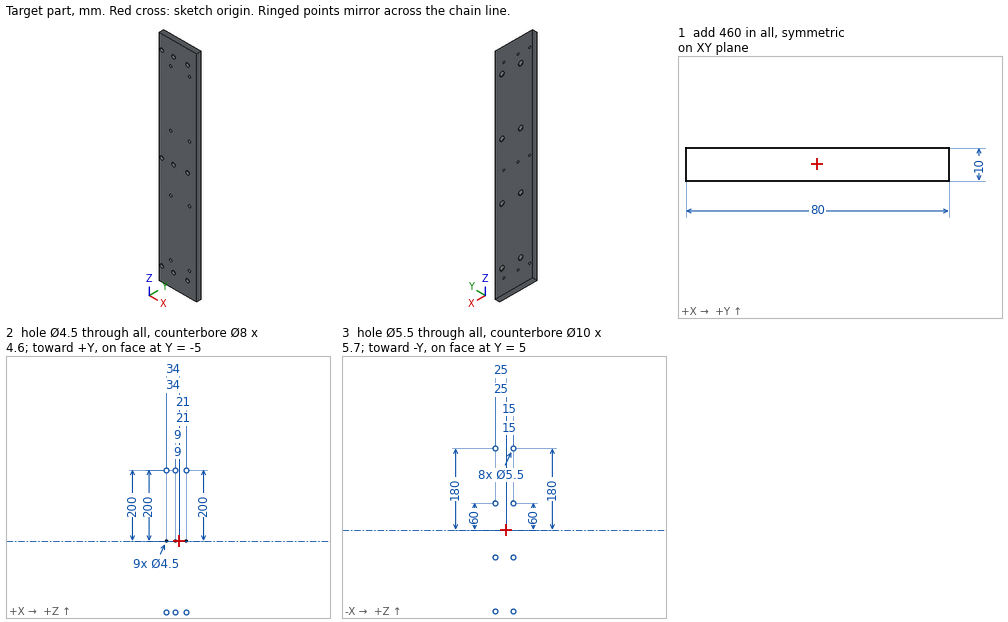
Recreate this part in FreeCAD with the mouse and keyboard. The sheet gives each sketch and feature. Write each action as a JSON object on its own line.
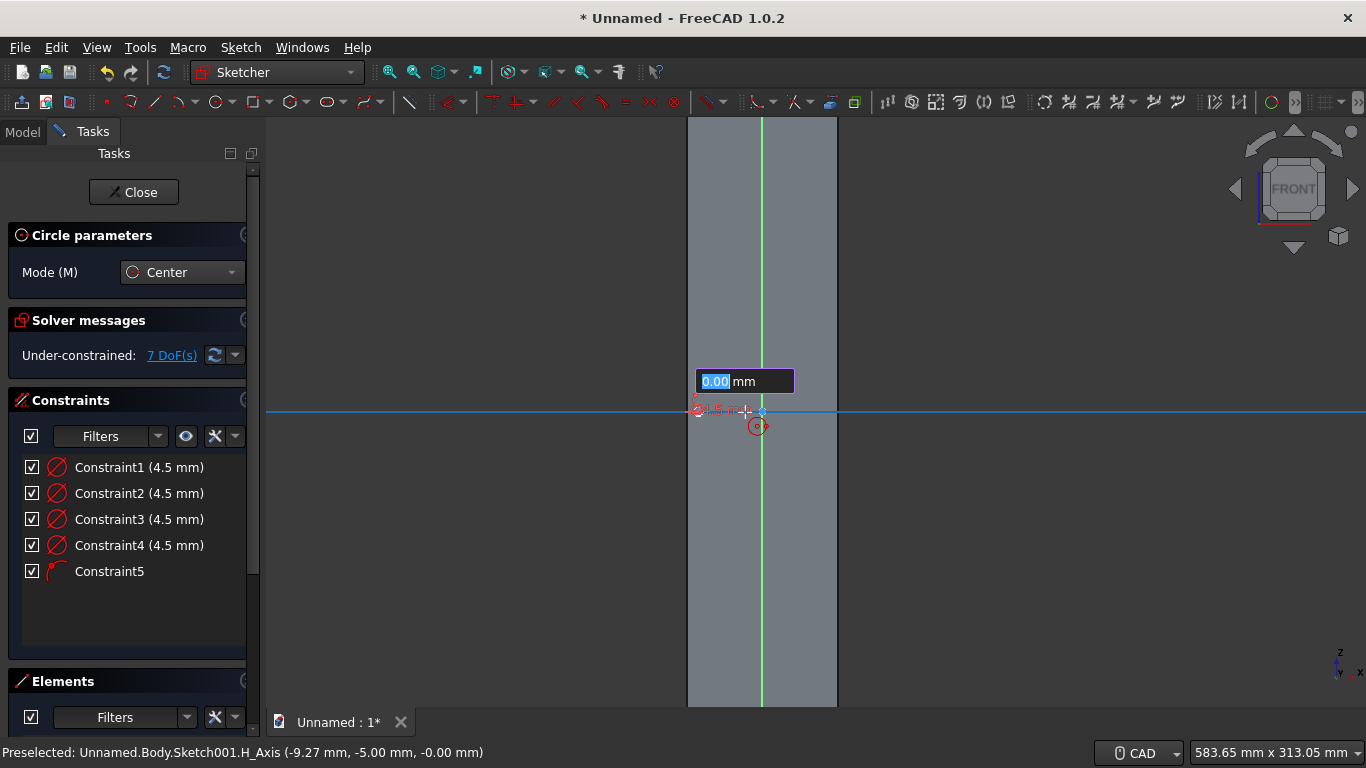
{"action": "scroll", "coordinate": [744, 416], "scroll_direction": "up", "scroll_amount": 7}
{"action": "mouse_move", "coordinate": [743, 414]}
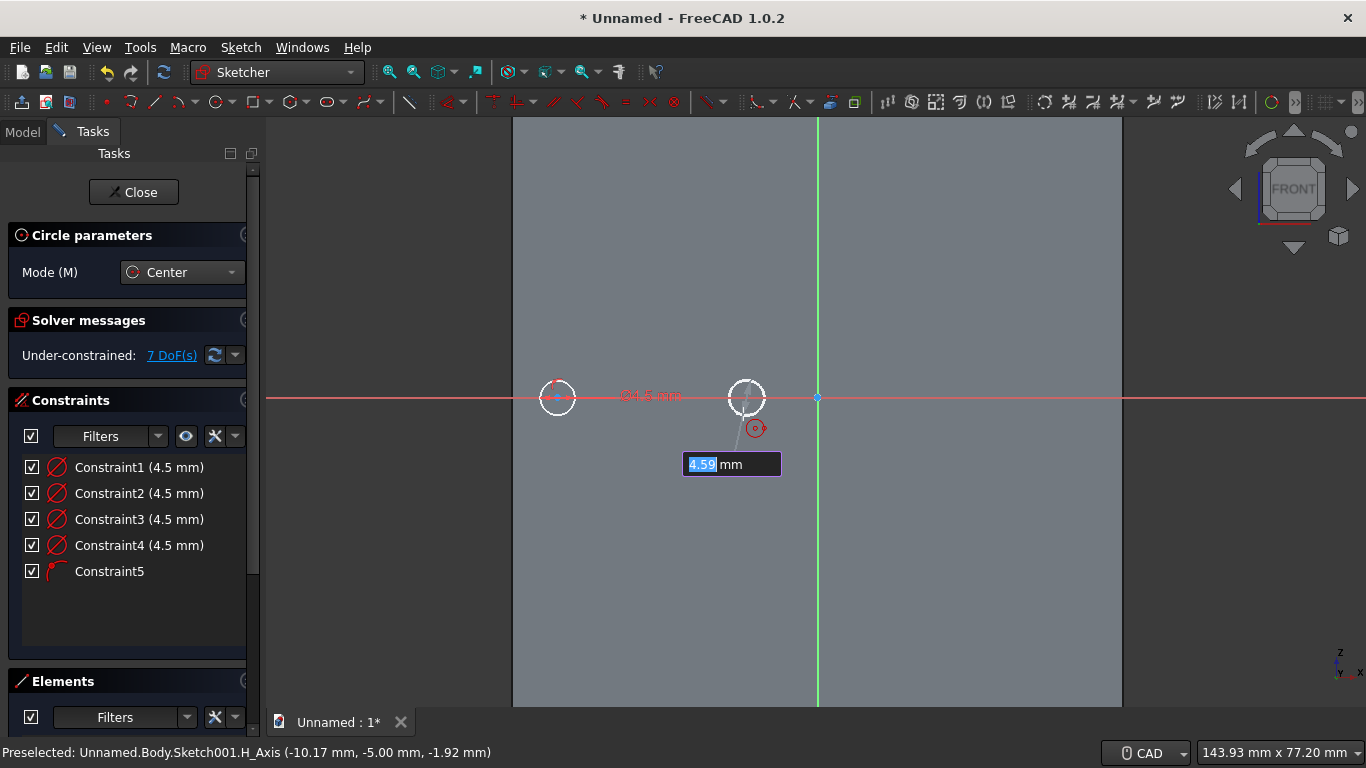
{"action": "type", "text": "4.5"}
{"action": "key", "text": "Return"}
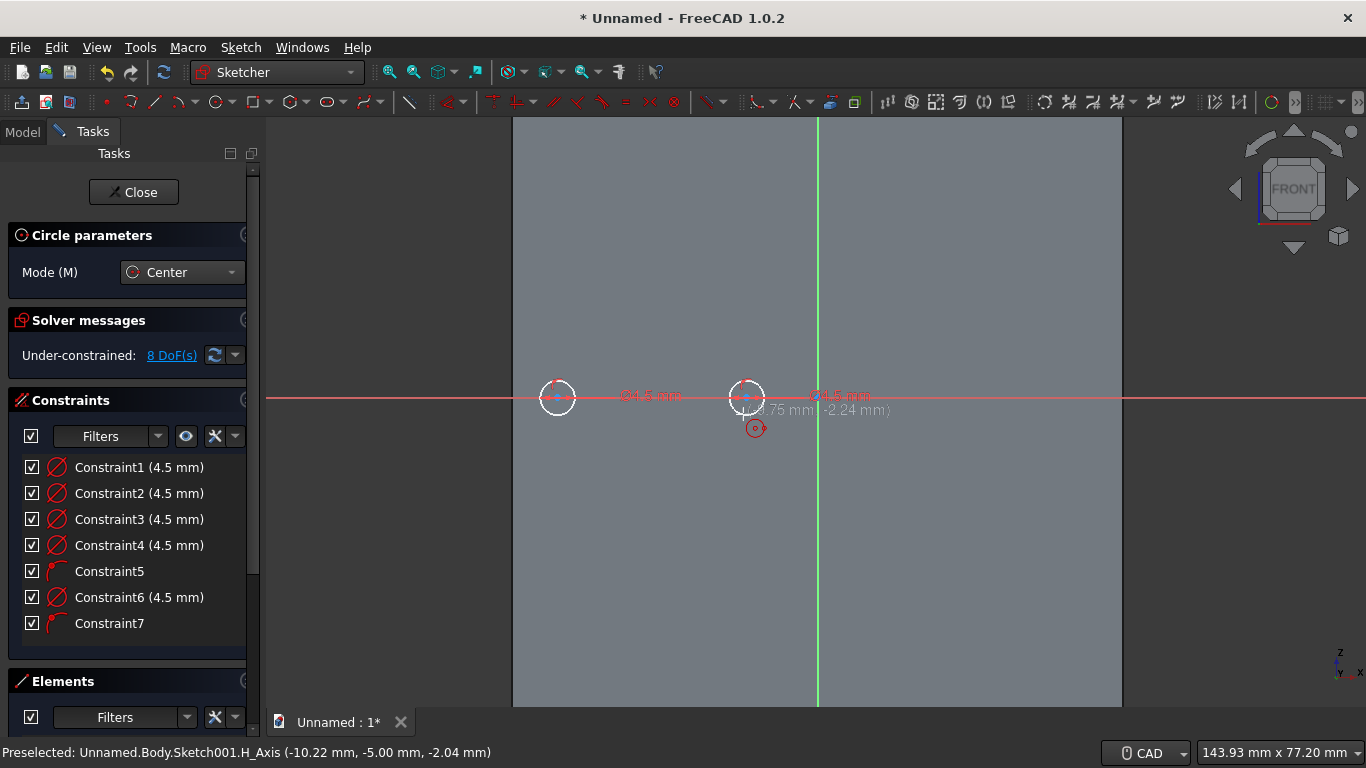
{"action": "scroll", "coordinate": [978, 398], "scroll_direction": "up", "scroll_amount": 2}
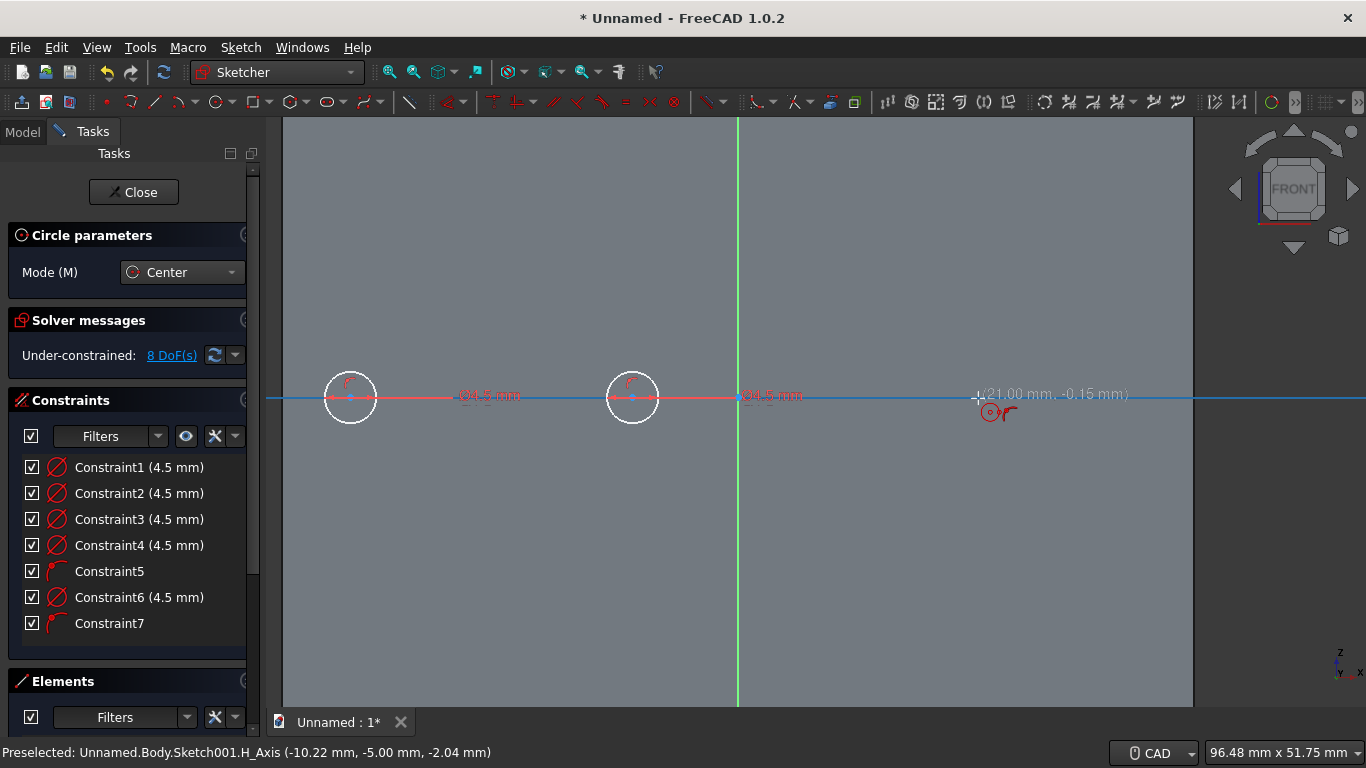
{"action": "scroll", "coordinate": [754, 413], "scroll_direction": "down", "scroll_amount": 13}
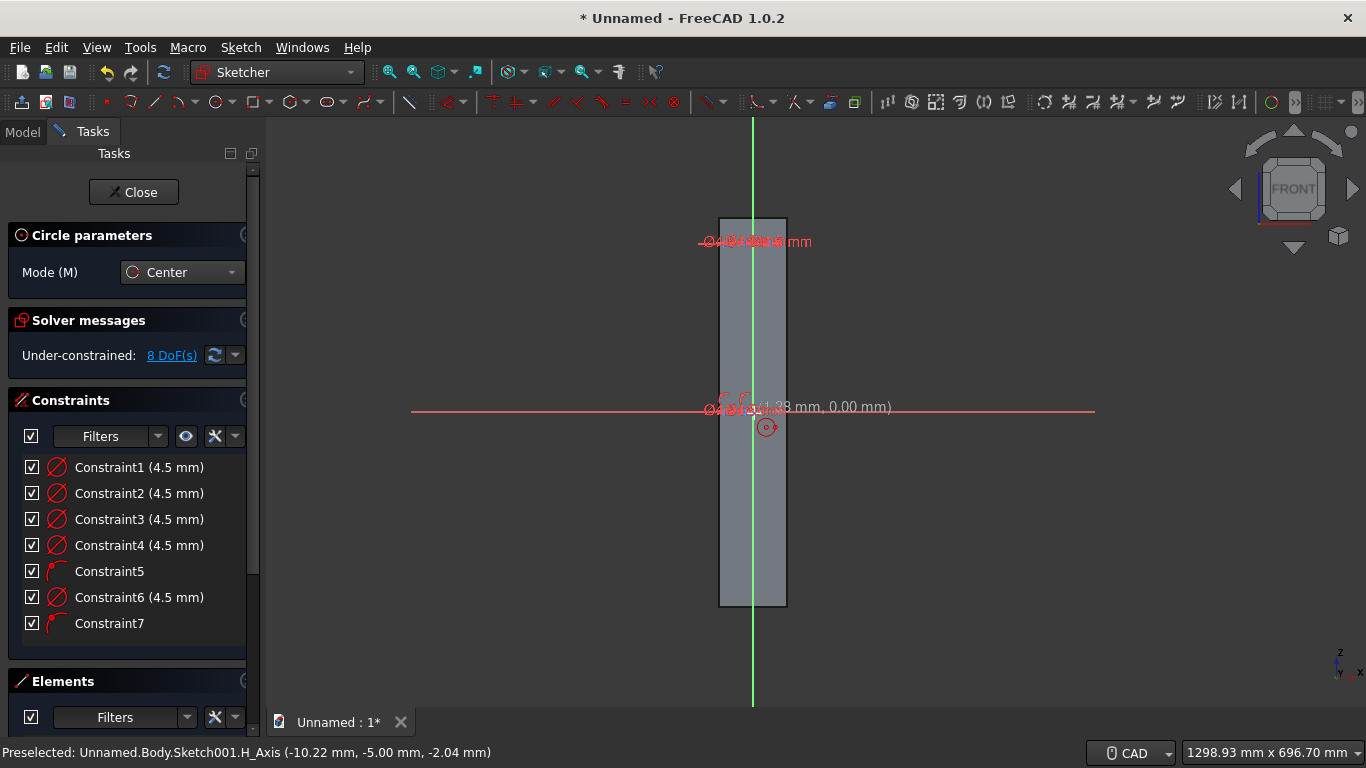
{"action": "left_click", "coordinate": [771, 412]}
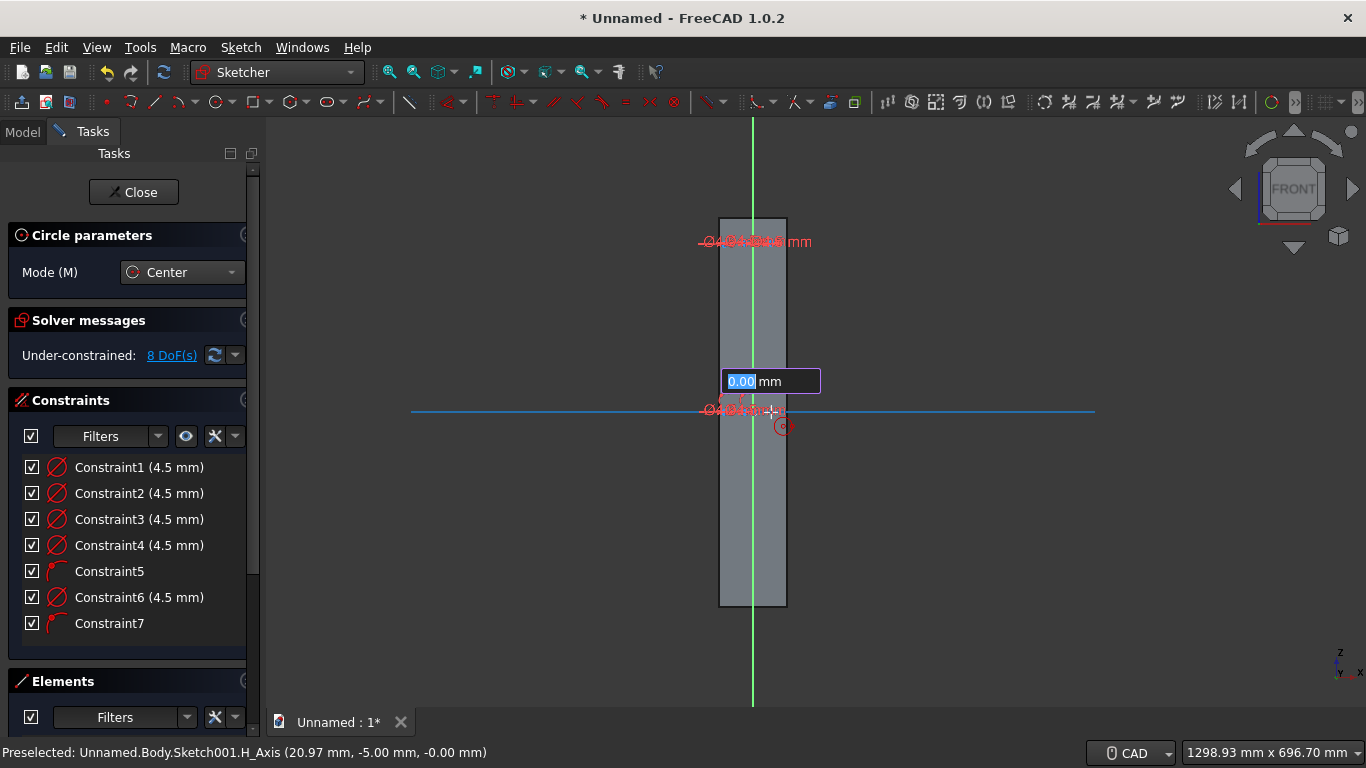
{"action": "scroll", "coordinate": [770, 414], "scroll_direction": "up", "scroll_amount": 11}
{"action": "mouse_move", "coordinate": [770, 411]}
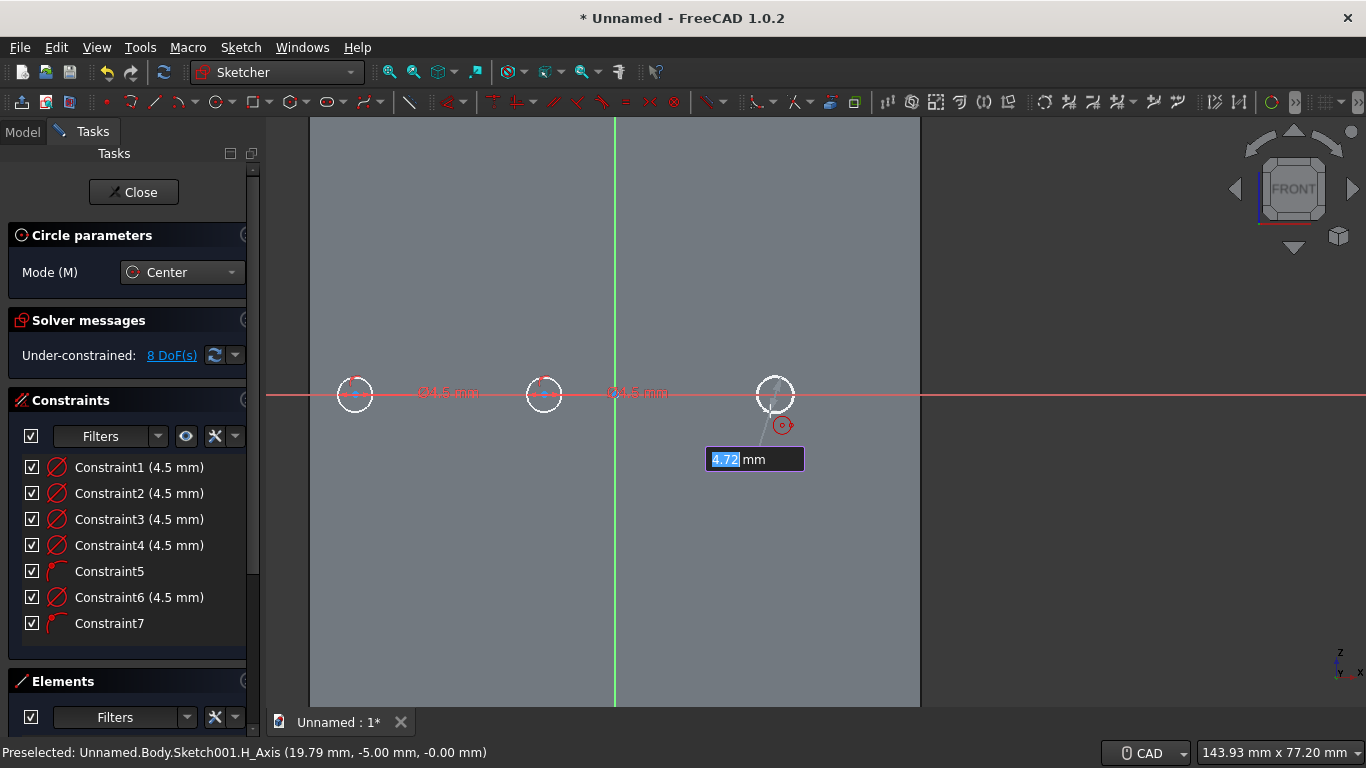
{"action": "type", "text": "4.5"}
{"action": "key", "text": "Return"}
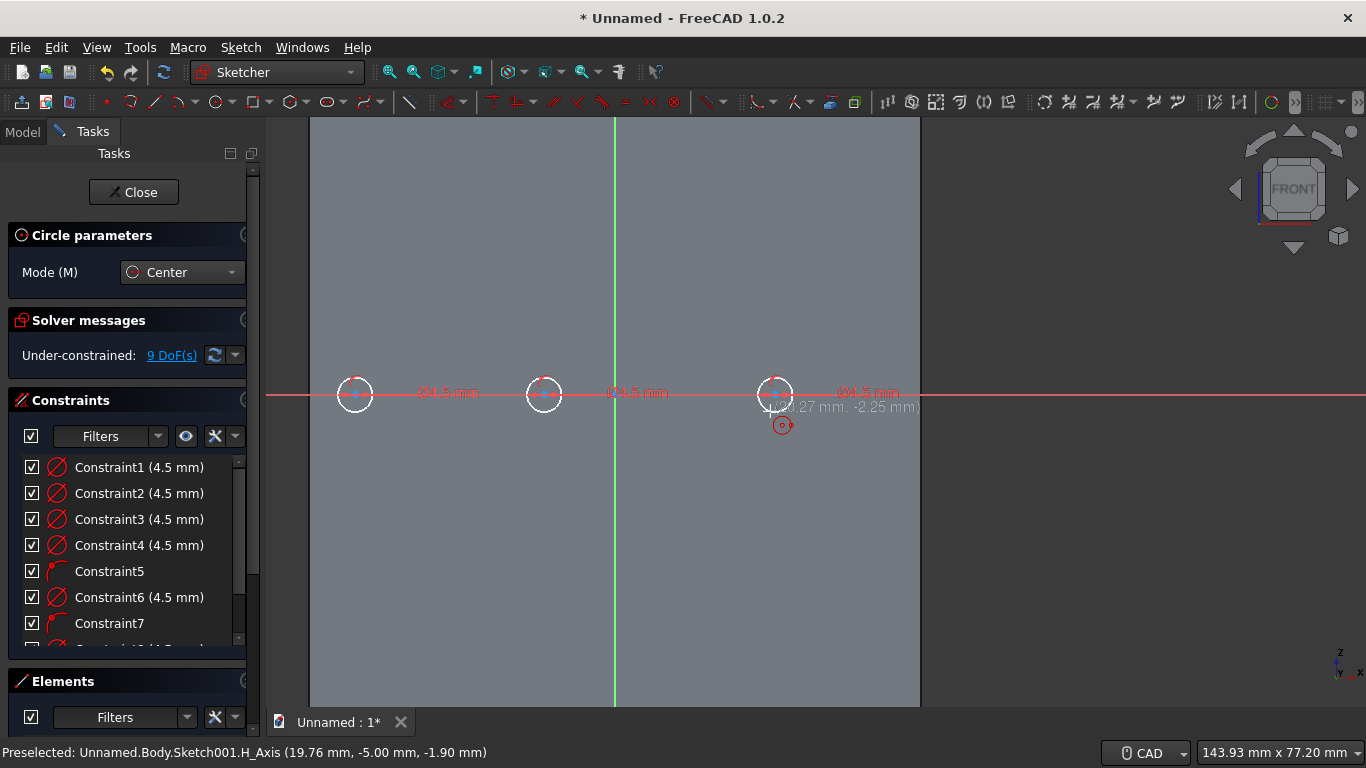
{"action": "scroll", "coordinate": [770, 414], "scroll_direction": "down", "scroll_amount": 11}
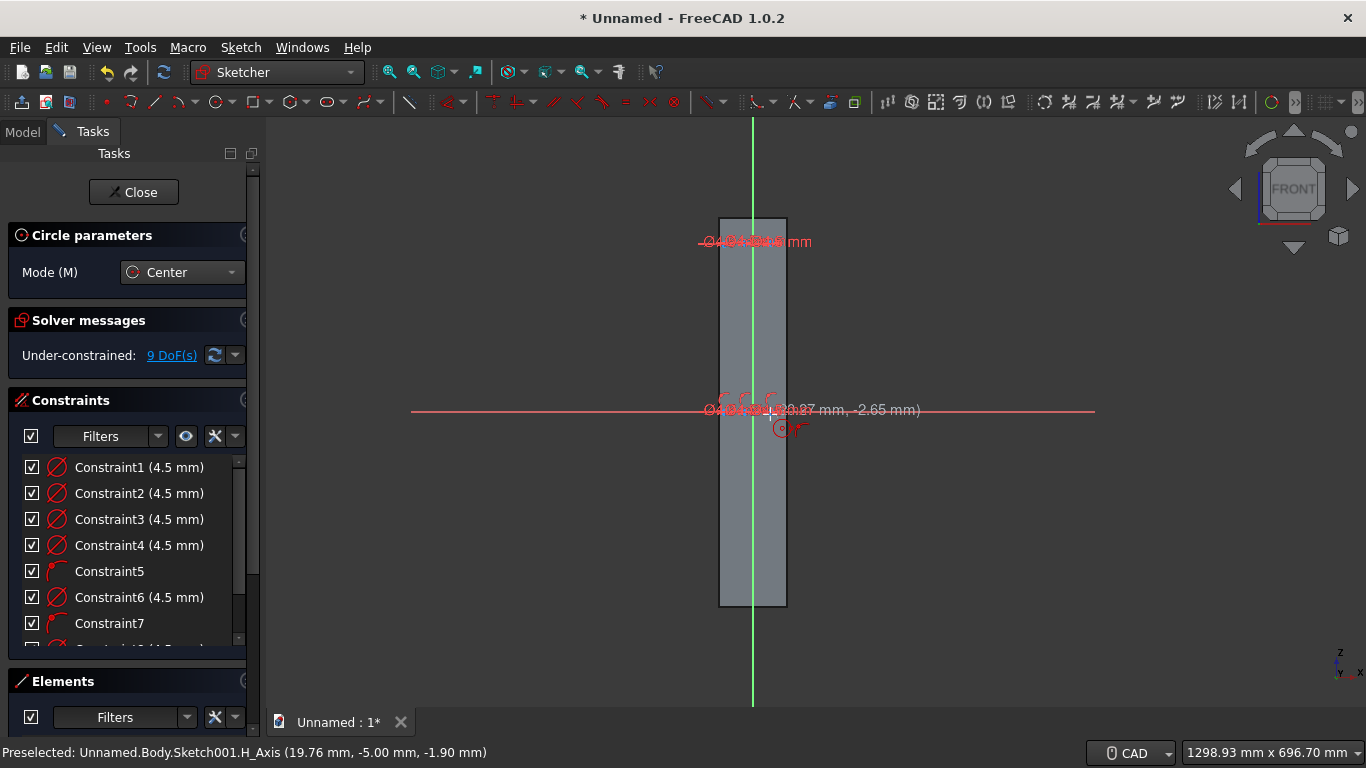
{"action": "scroll", "coordinate": [724, 582], "scroll_direction": "up", "scroll_amount": 13}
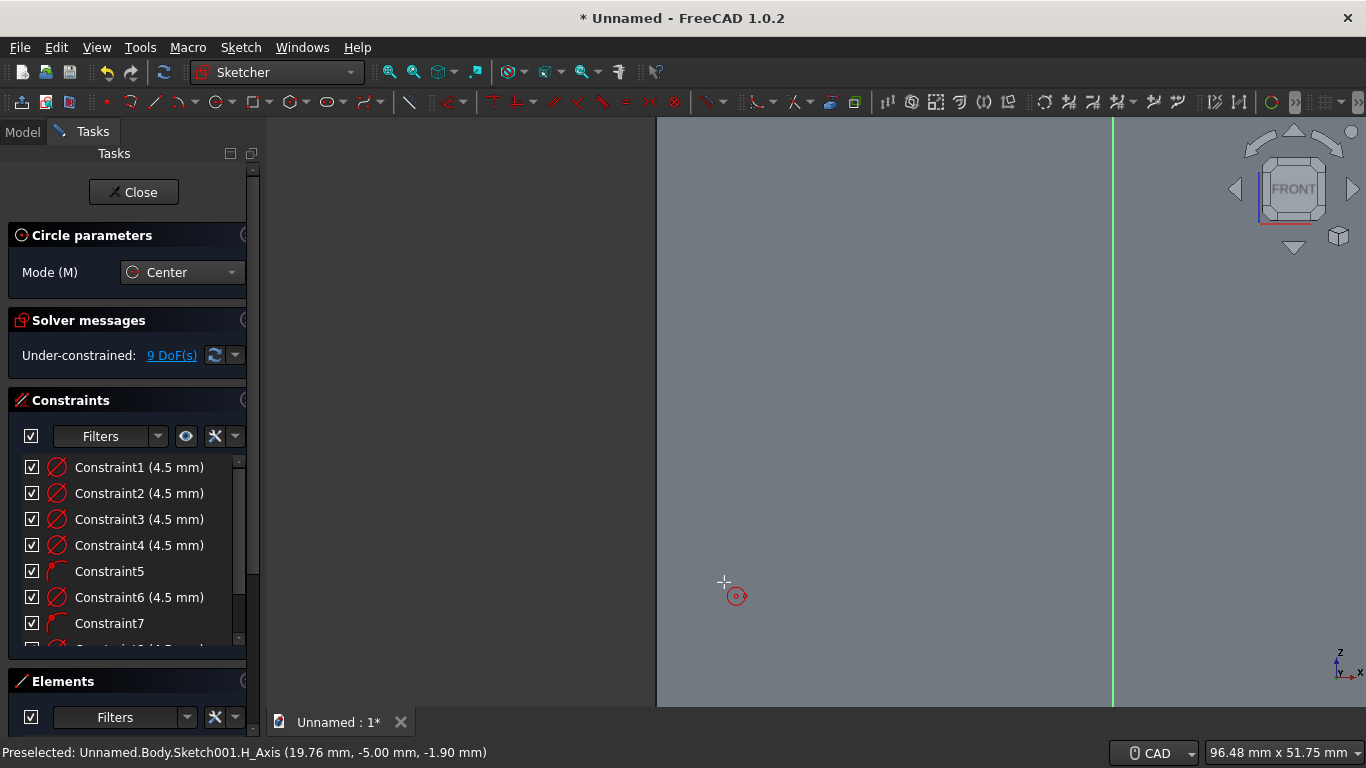
{"action": "scroll", "coordinate": [724, 582], "scroll_direction": "down", "scroll_amount": 13}